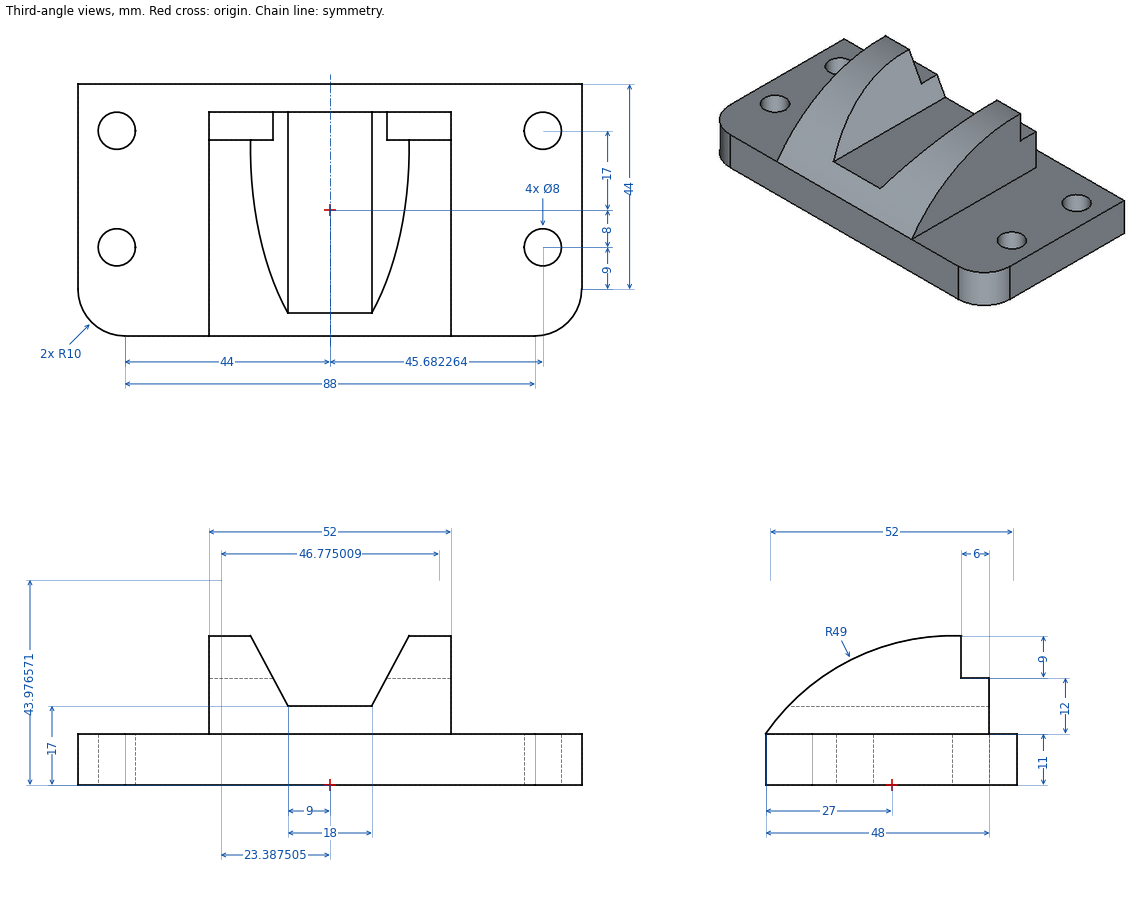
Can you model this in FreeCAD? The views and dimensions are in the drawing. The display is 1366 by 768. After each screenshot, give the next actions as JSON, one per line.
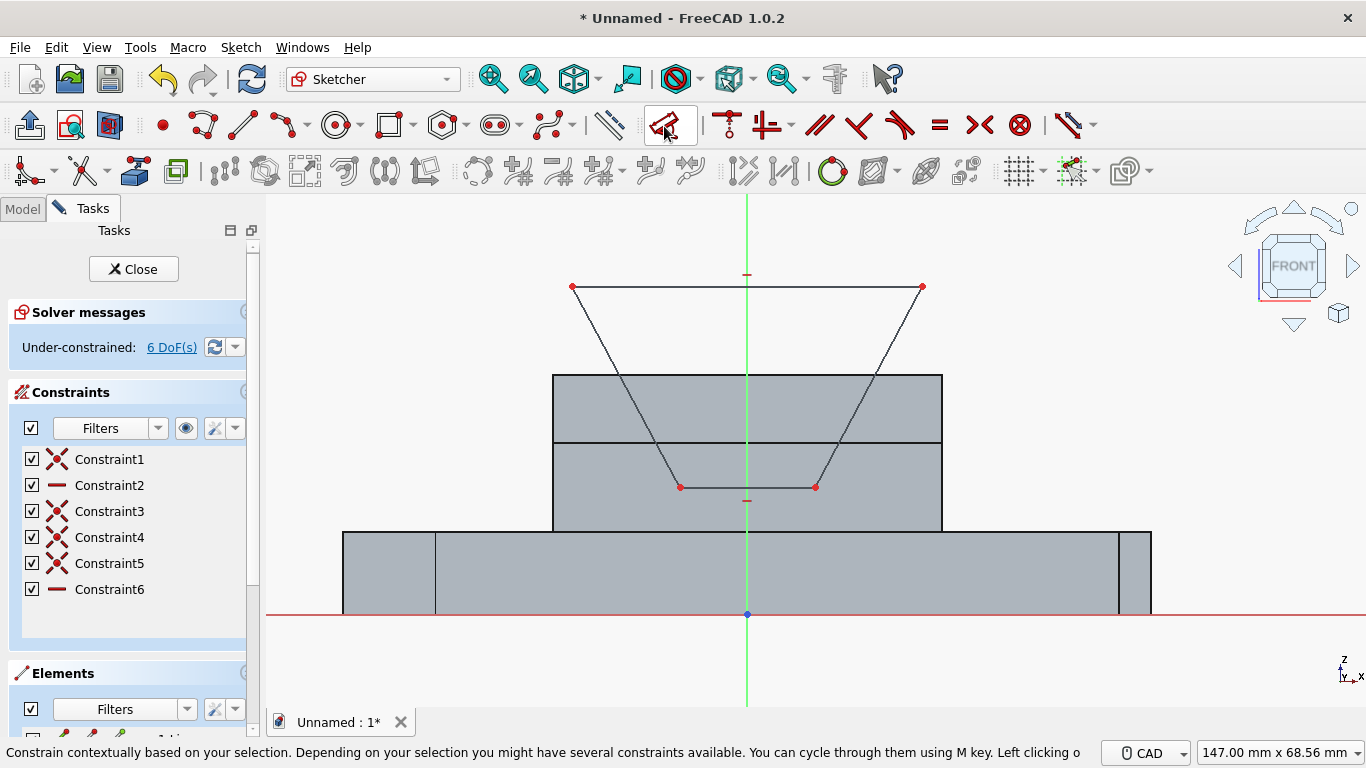
{"action": "left_click", "coordinate": [775, 488]}
{"action": "left_click", "coordinate": [716, 522]}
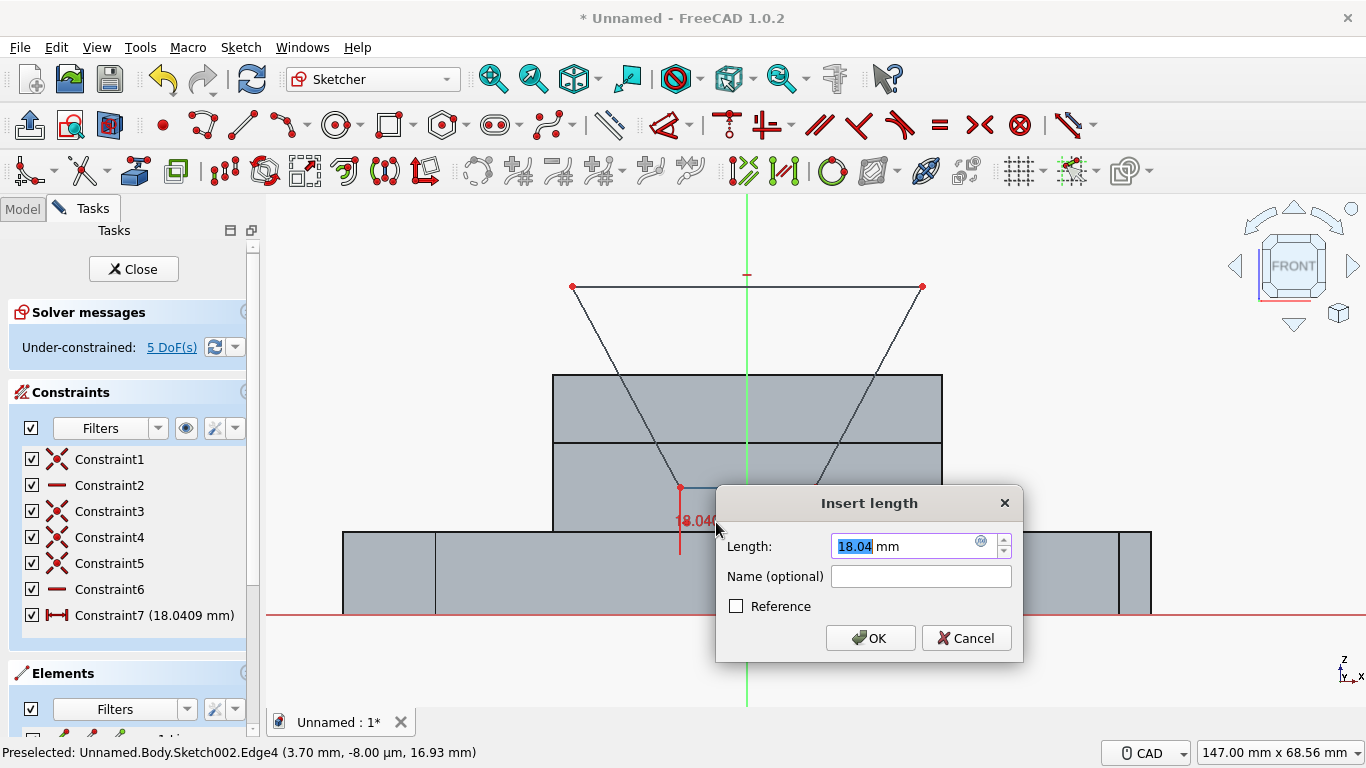
{"action": "type", "text": "18"}
{"action": "key", "text": "Return"}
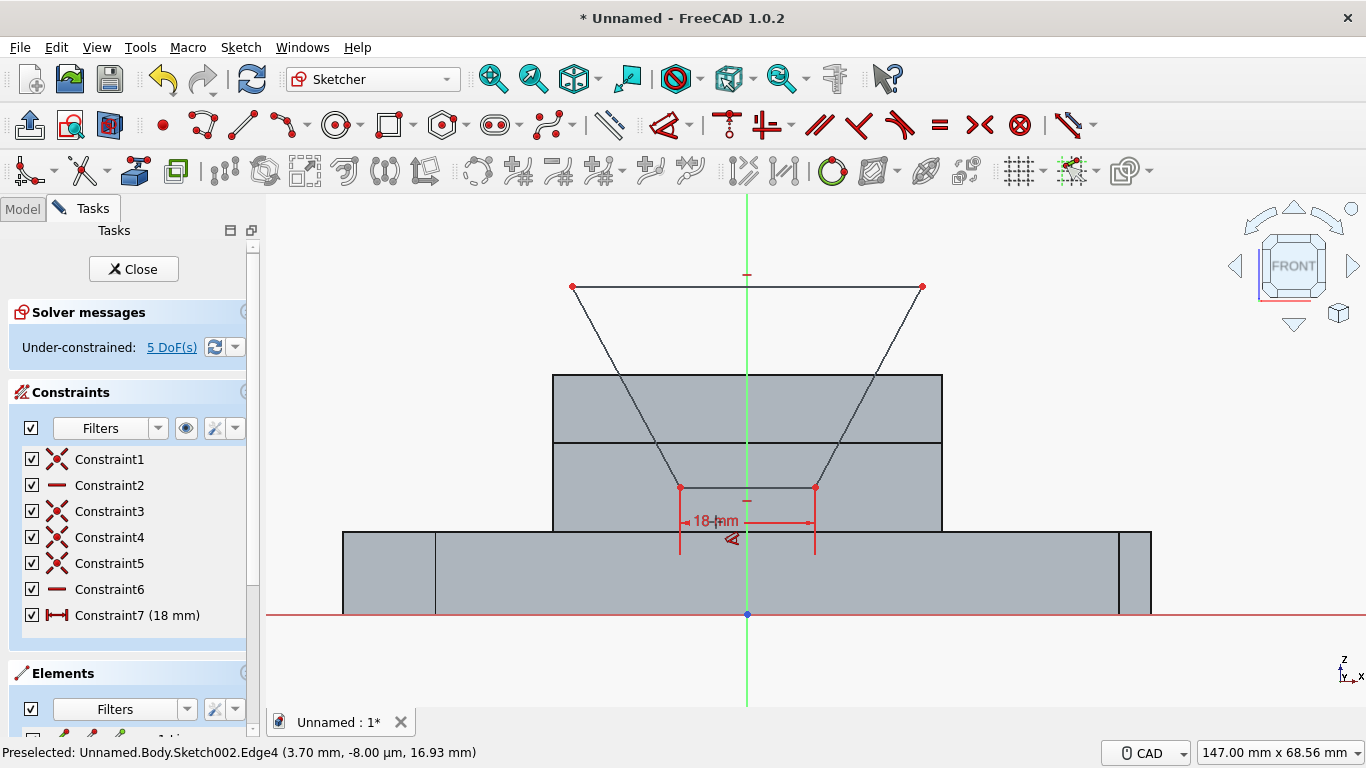
{"action": "left_click", "coordinate": [680, 488]}
{"action": "left_click", "coordinate": [714, 649]}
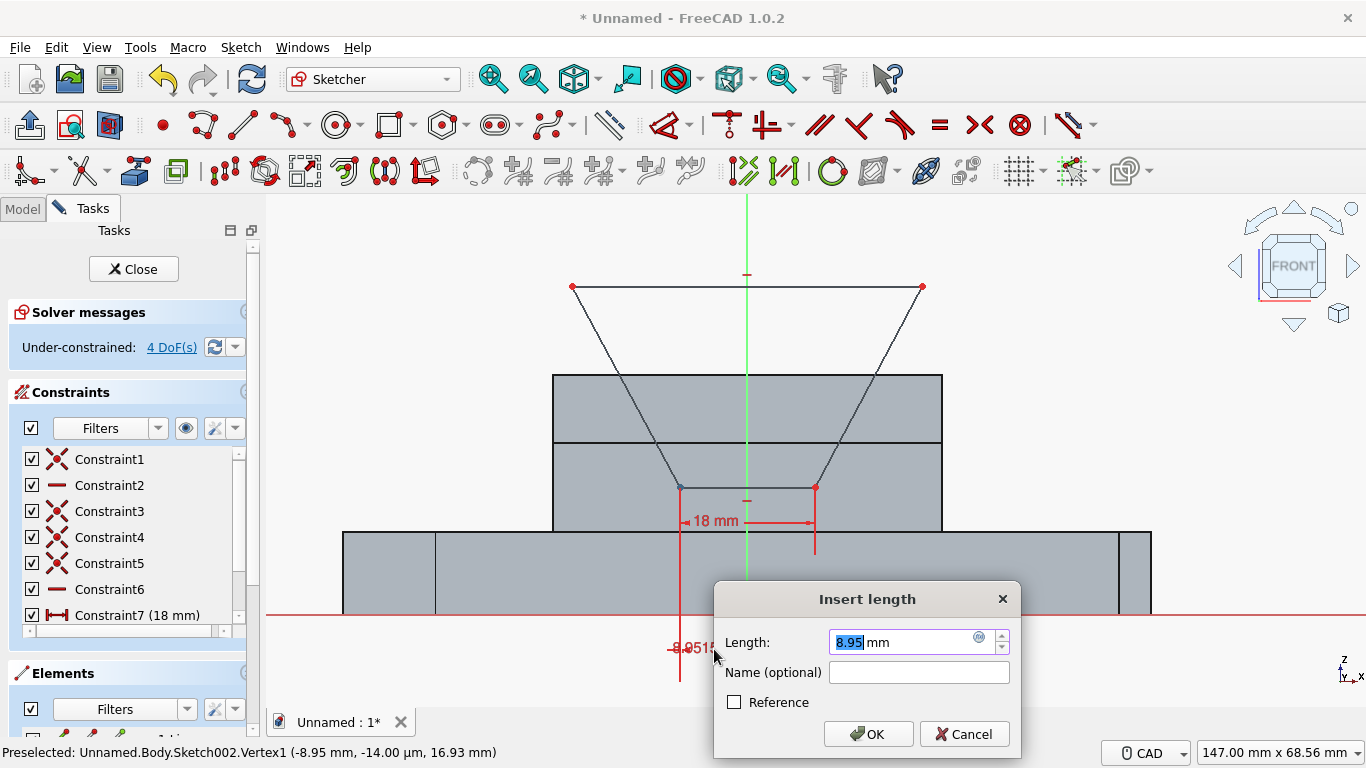
{"action": "type", "text": "9"}
{"action": "key", "text": "Return"}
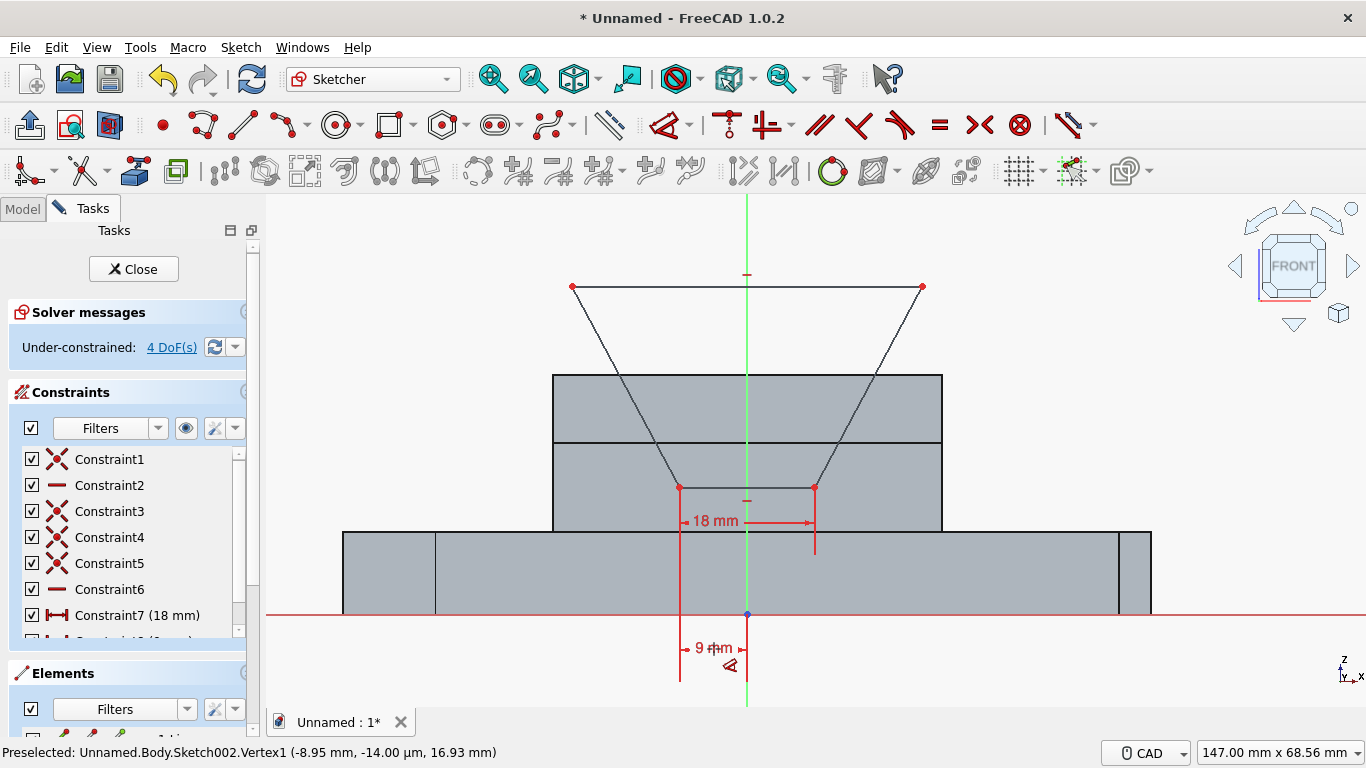
{"action": "left_click", "coordinate": [680, 488]}
{"action": "left_click", "coordinate": [646, 551]}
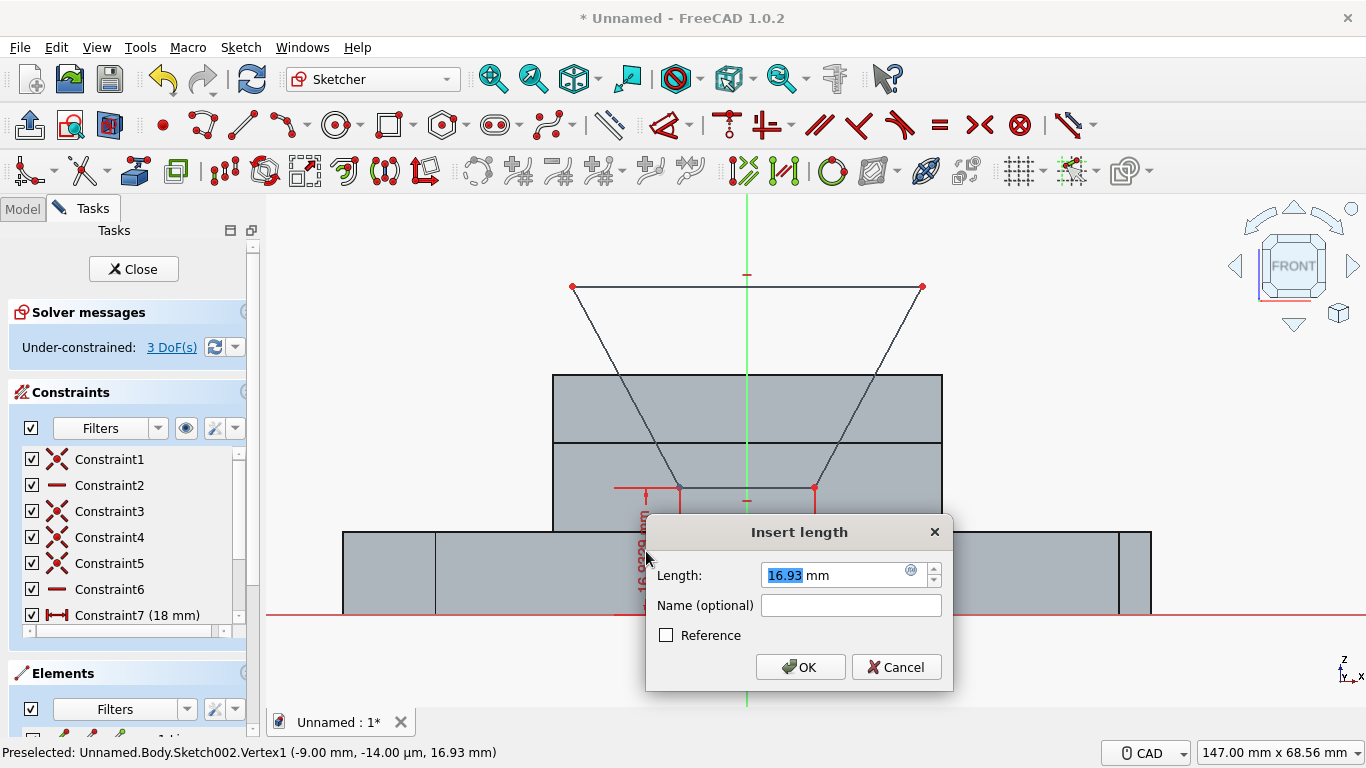
{"action": "type", "text": "17"}
{"action": "key", "text": "Return"}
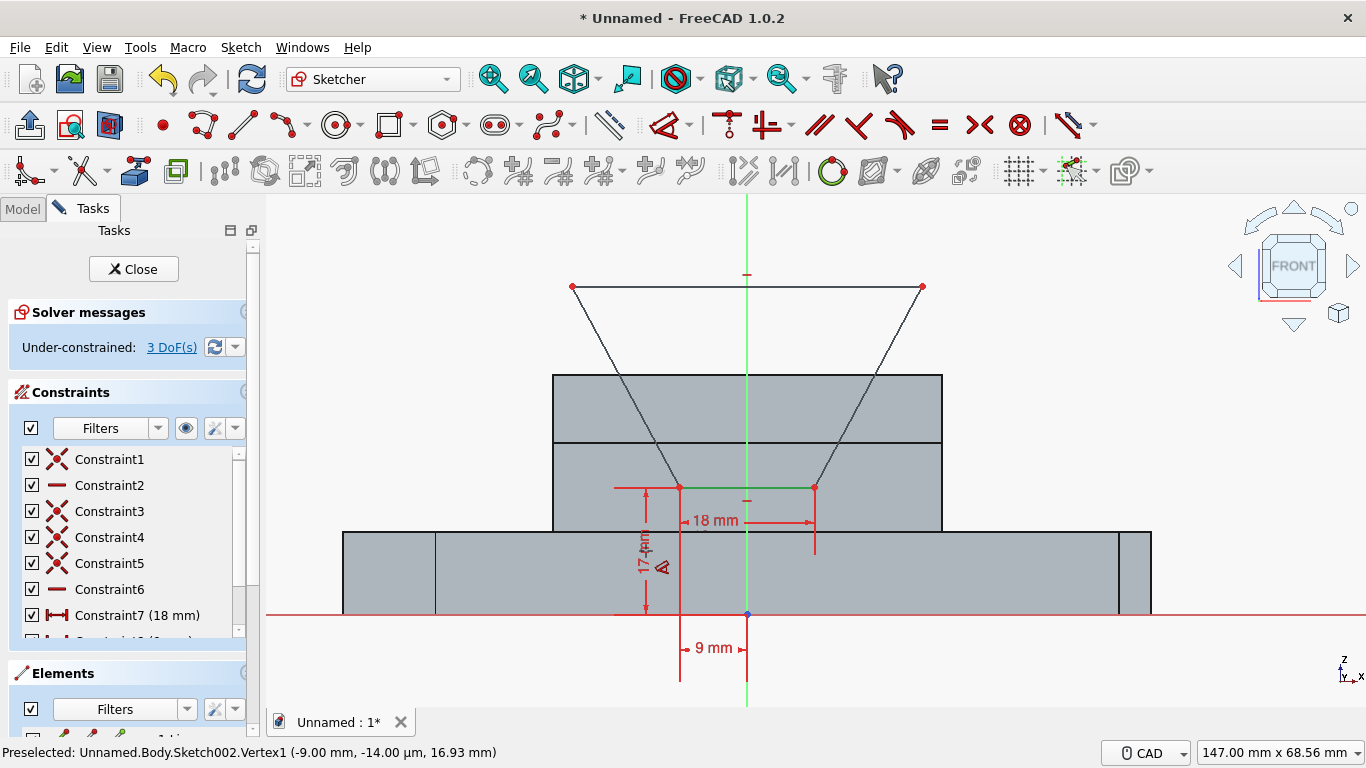
{"action": "left_click", "coordinate": [677, 287]}
{"action": "left_click", "coordinate": [667, 253]}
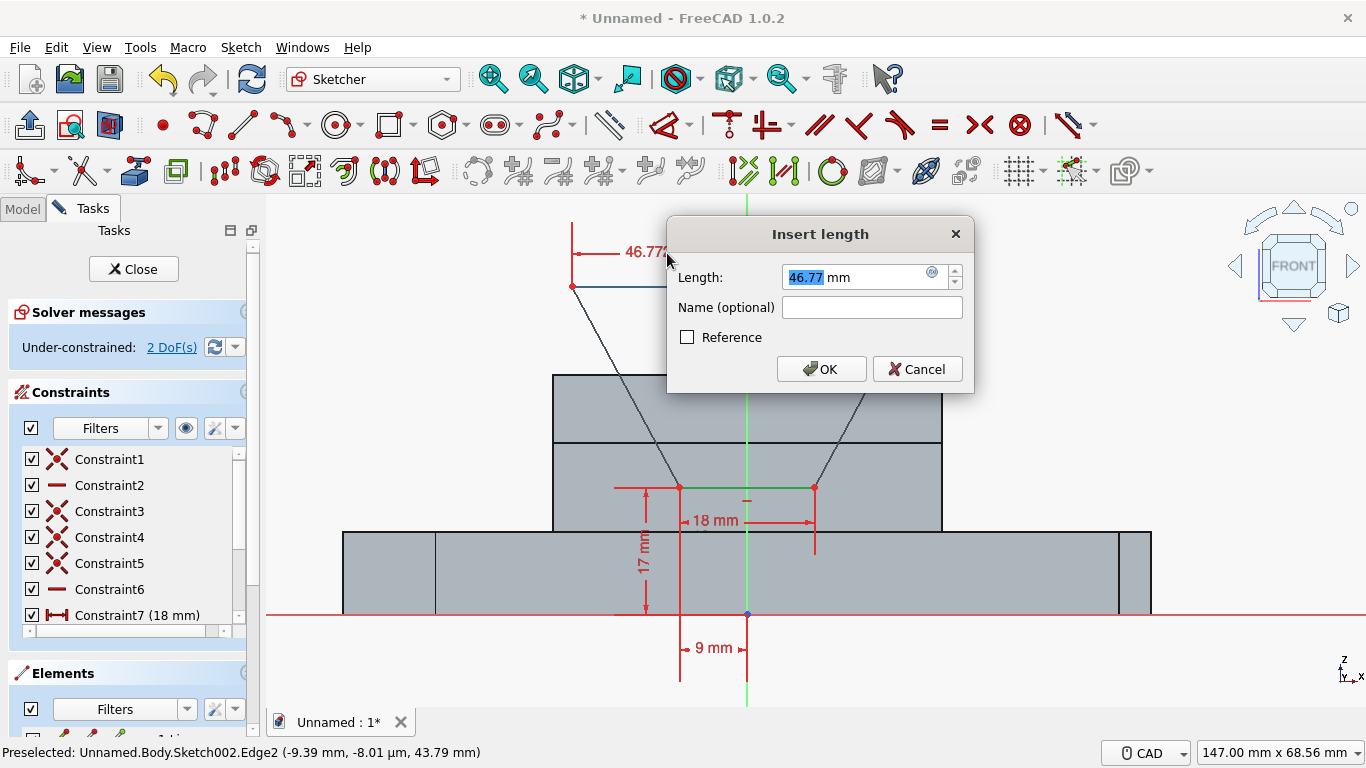
{"action": "type", "text": "46.775009"}
{"action": "key", "text": "Return"}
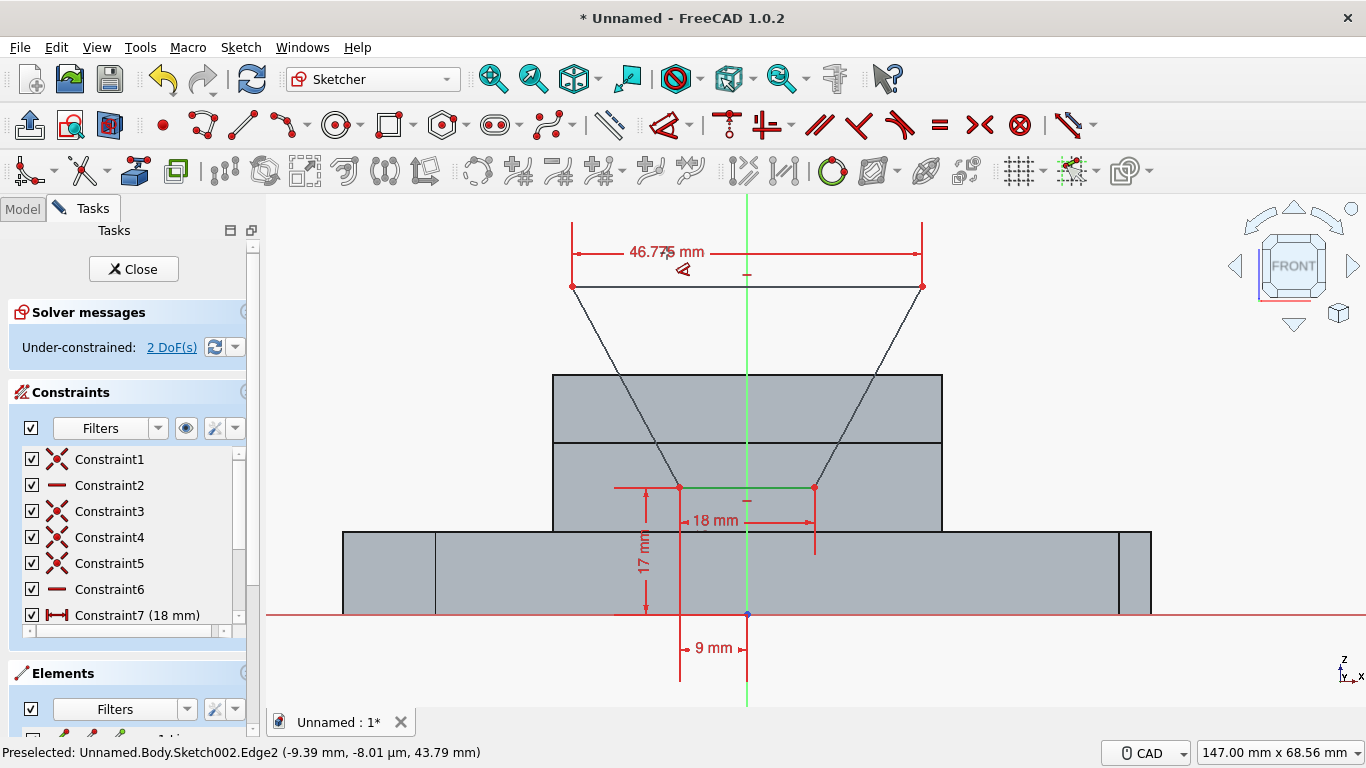
{"action": "left_click", "coordinate": [572, 287]}
{"action": "left_click", "coordinate": [619, 649]}